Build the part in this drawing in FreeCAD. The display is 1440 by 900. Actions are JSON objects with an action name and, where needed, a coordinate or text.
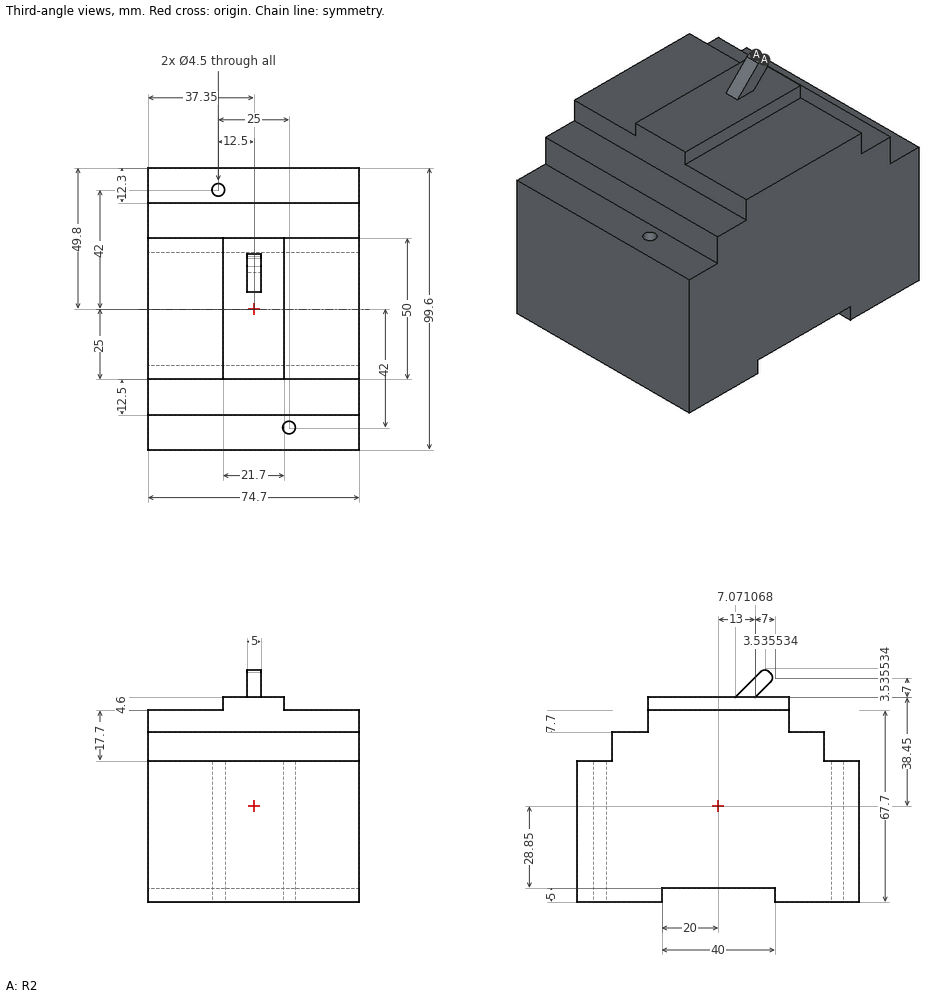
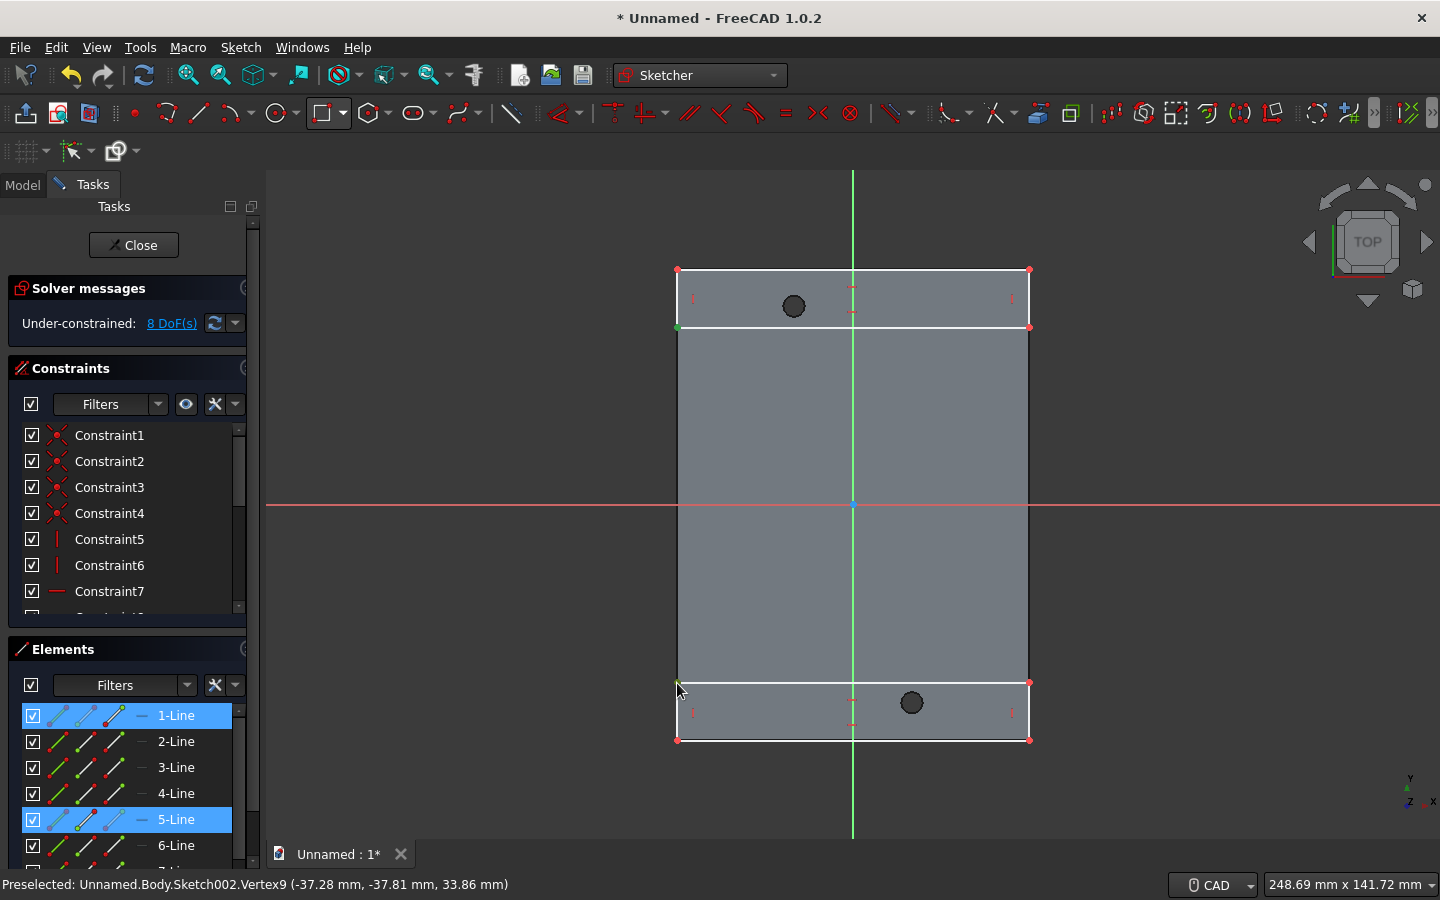
{"action": "left_click", "coordinate": [364, 504]}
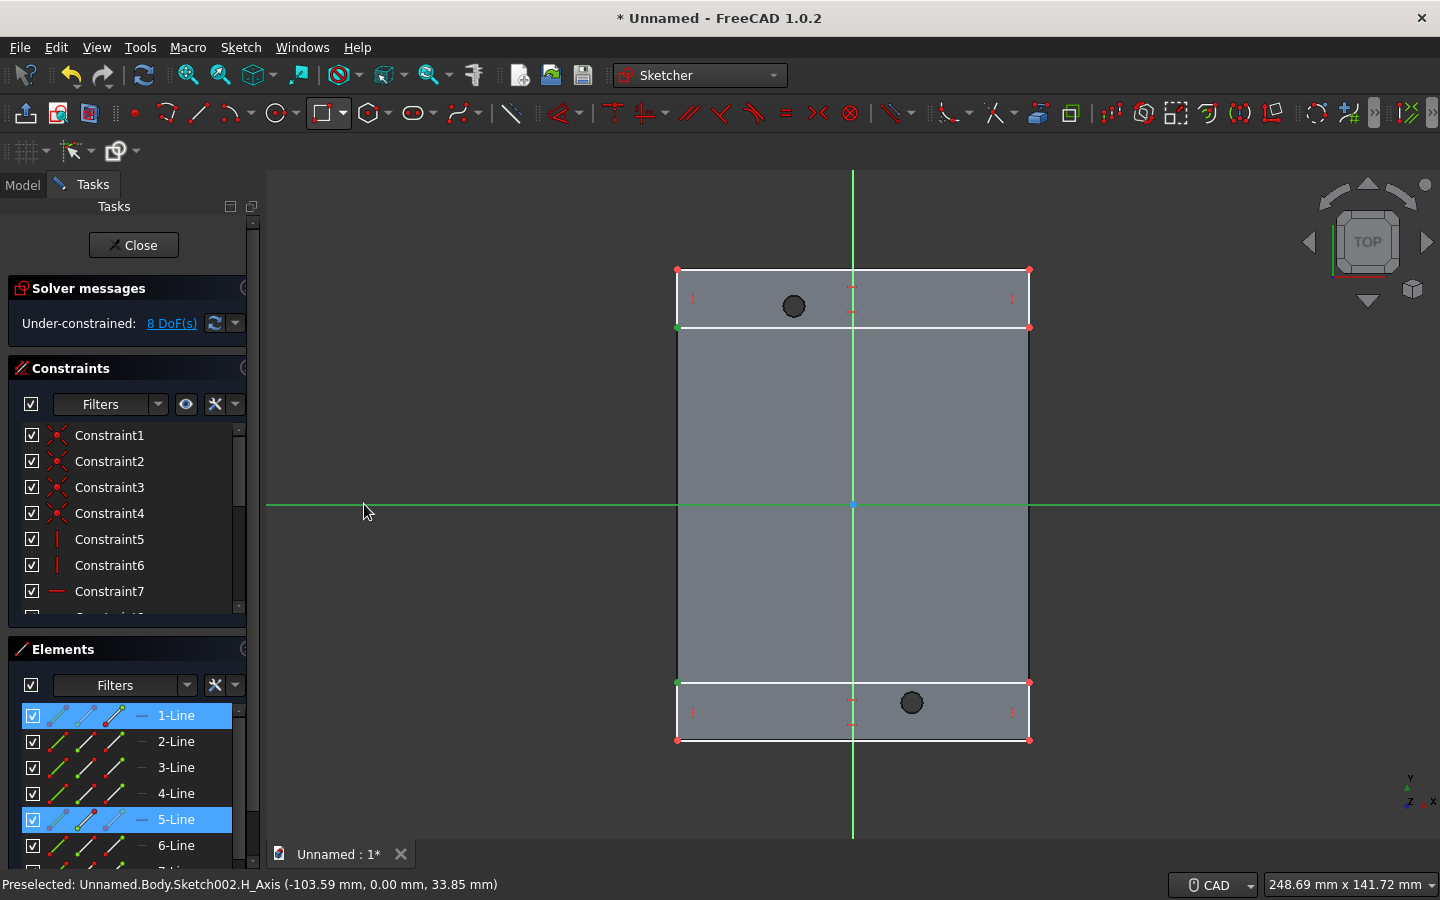
{"action": "key", "text": "s"}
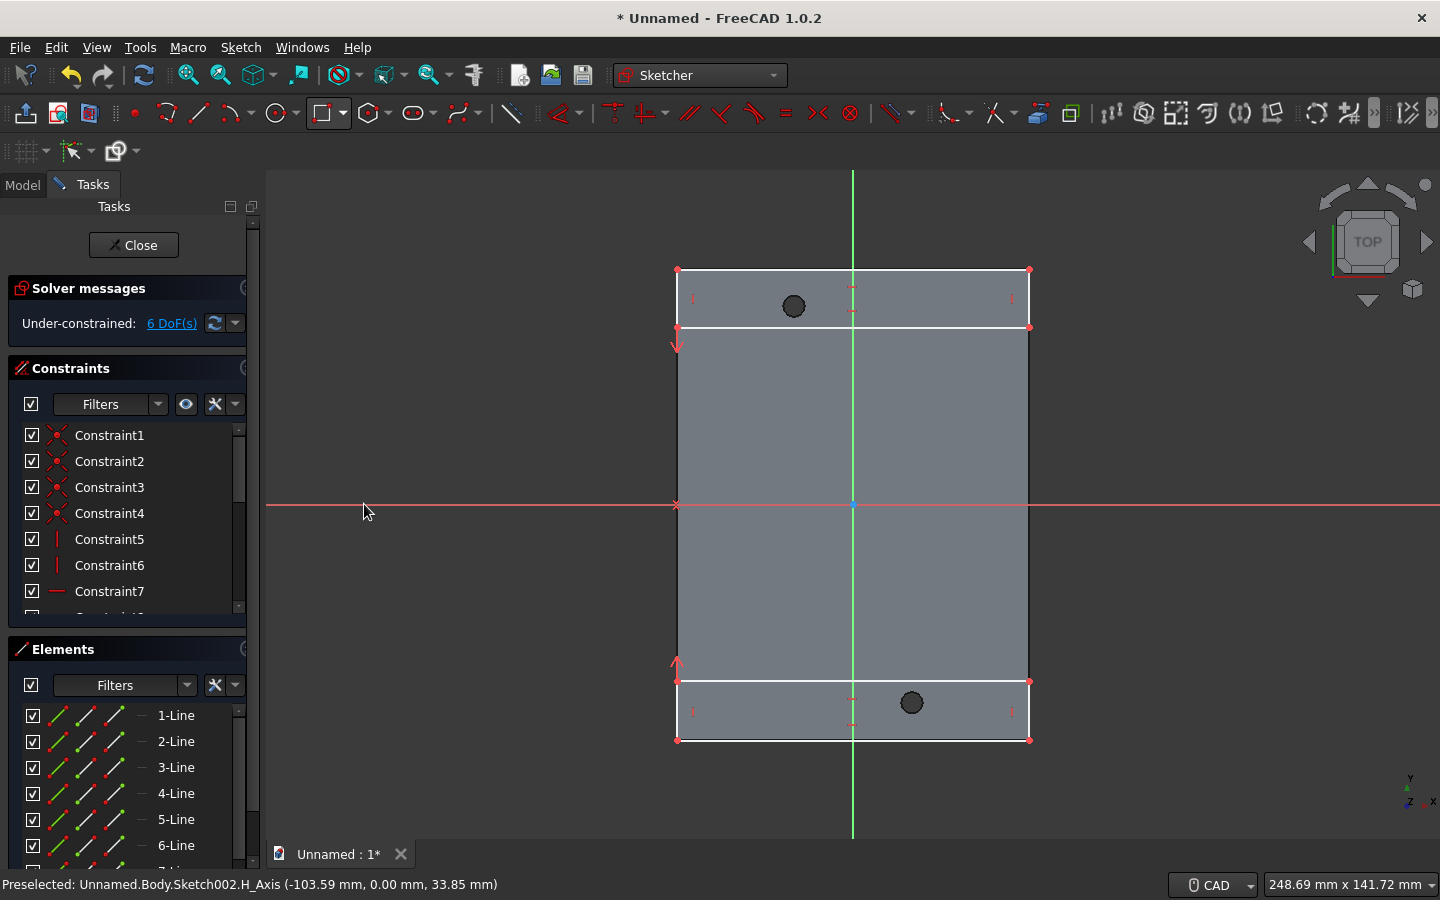
{"action": "left_click", "coordinate": [1029, 270]}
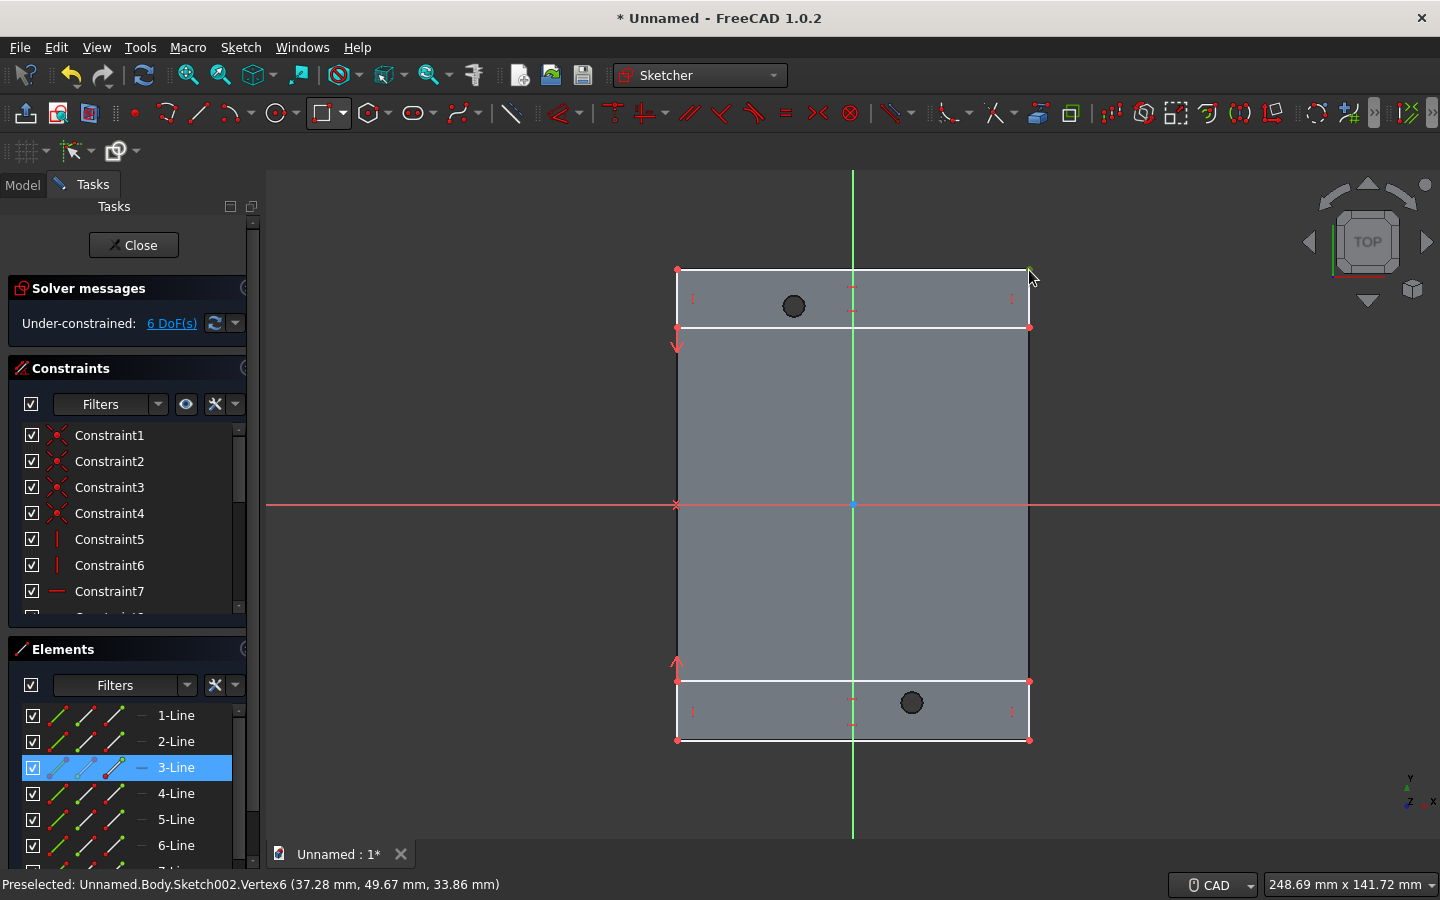
{"action": "left_click", "coordinate": [1029, 741]}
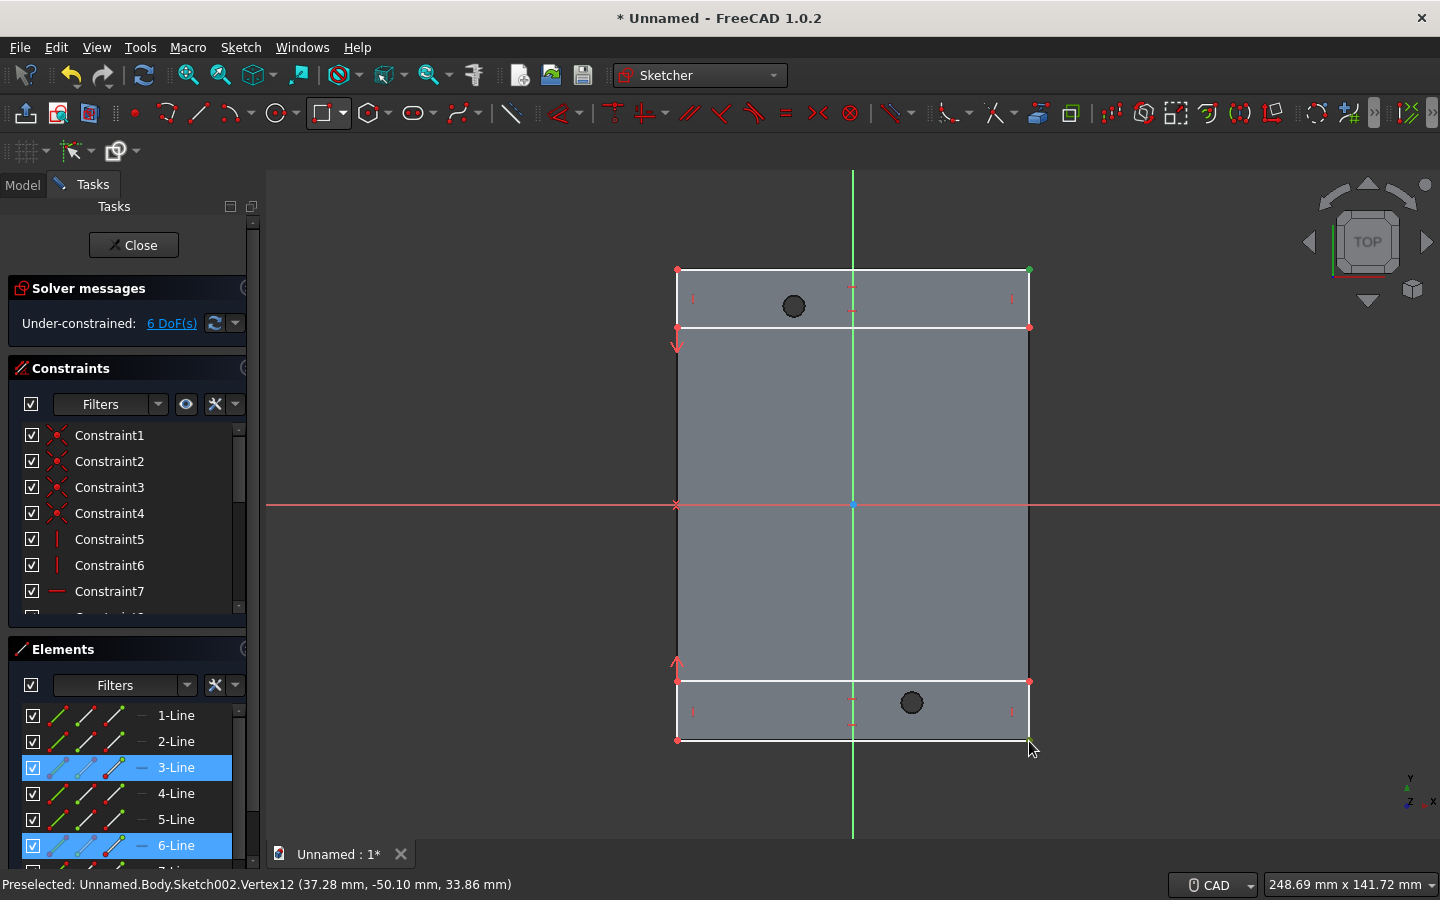
{"action": "left_click", "coordinate": [364, 504]}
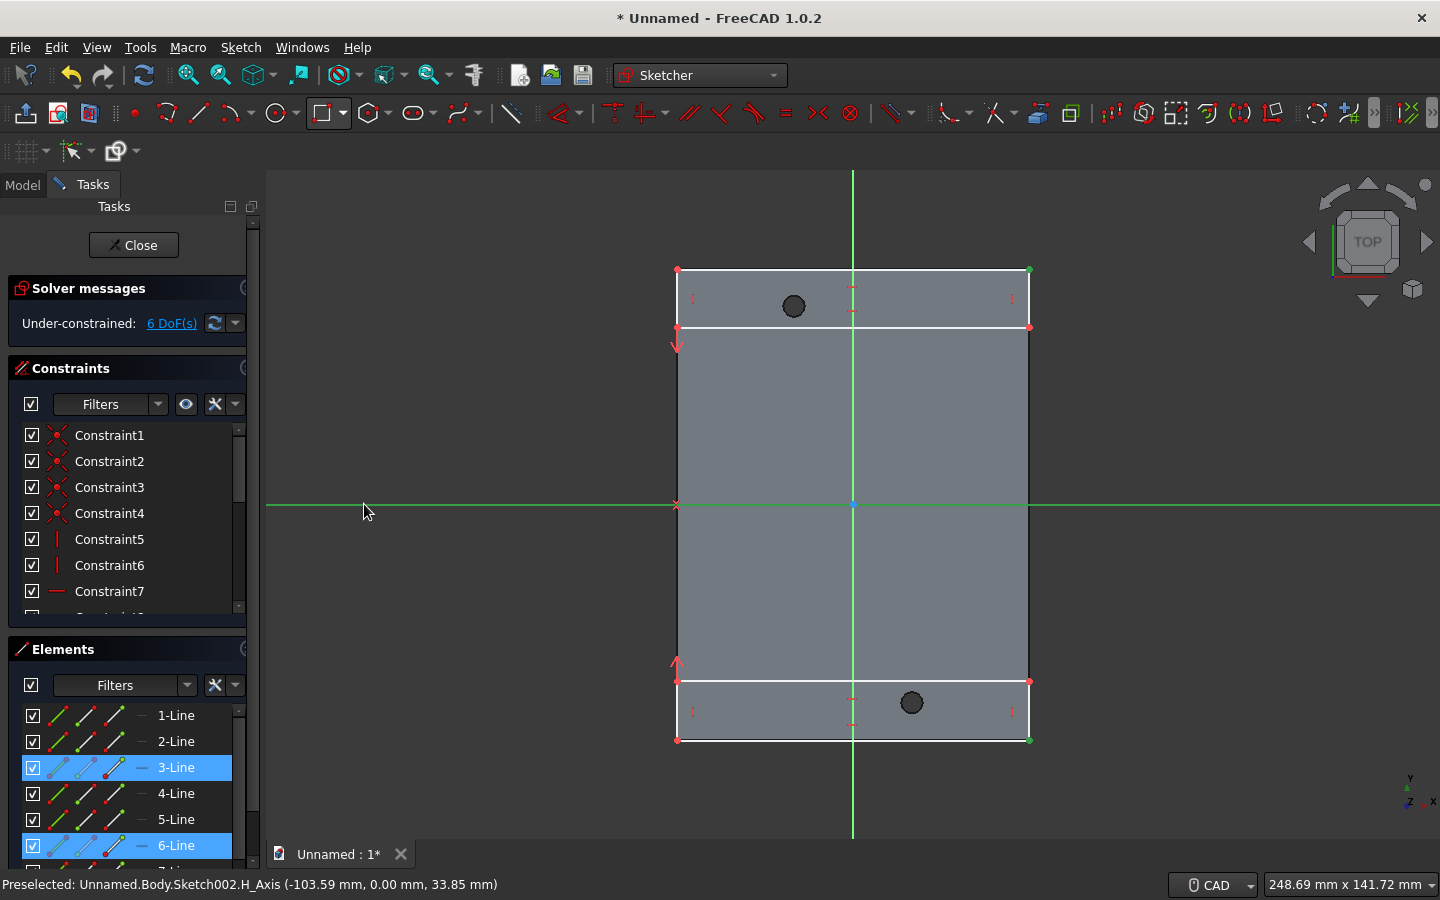
{"action": "left_click", "coordinate": [818, 114]}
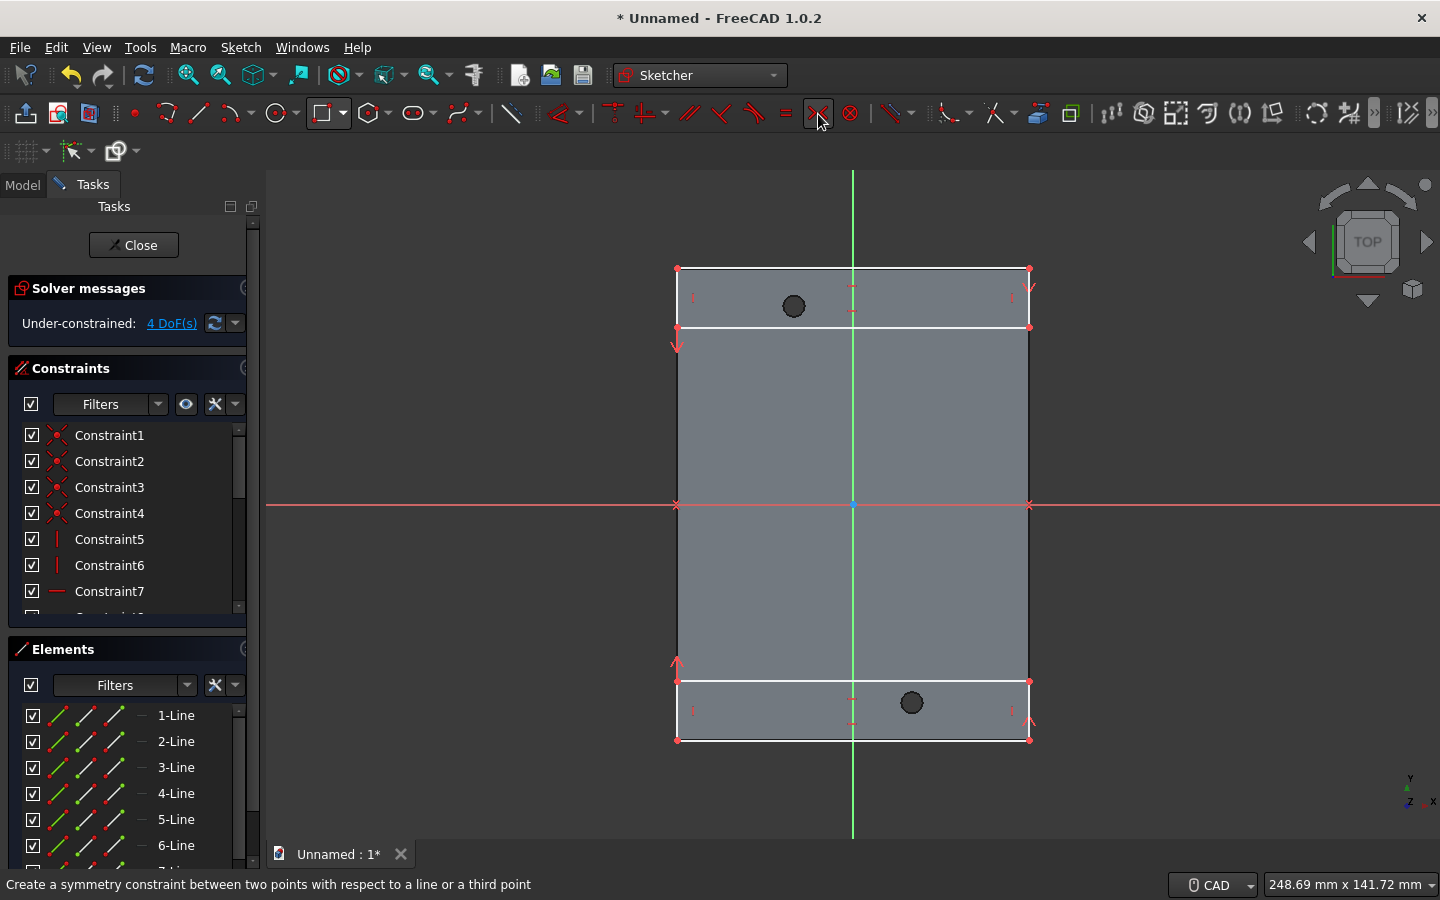
{"action": "left_click", "coordinate": [558, 114]}